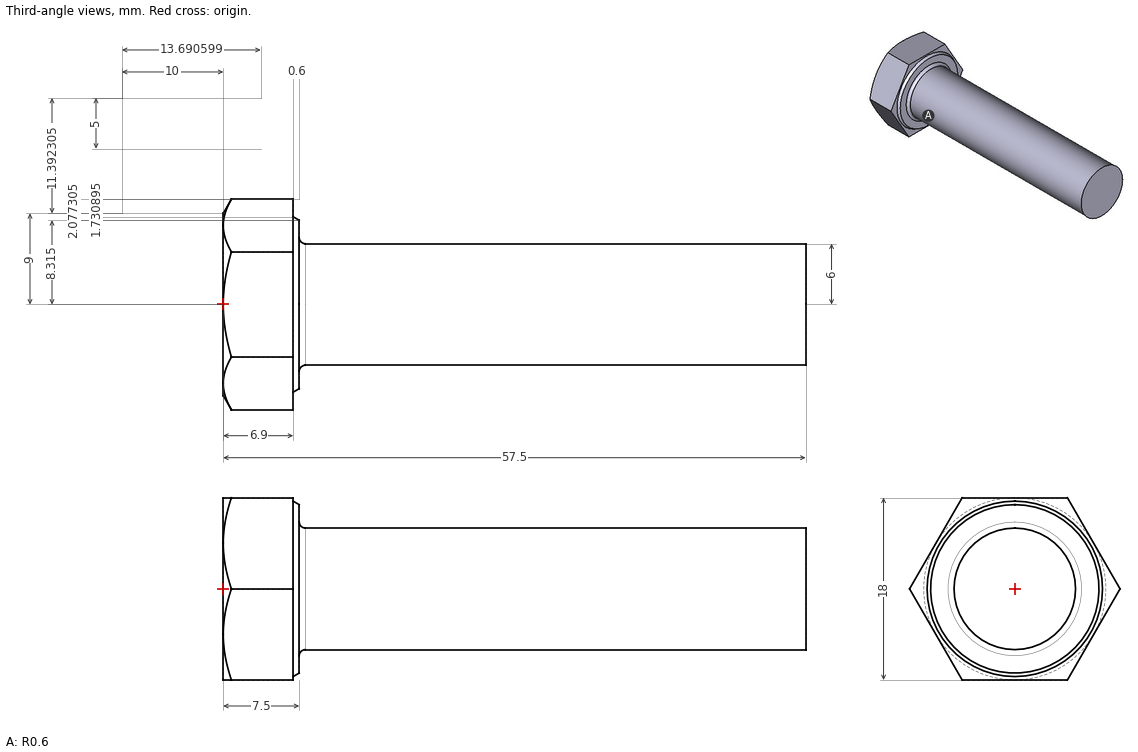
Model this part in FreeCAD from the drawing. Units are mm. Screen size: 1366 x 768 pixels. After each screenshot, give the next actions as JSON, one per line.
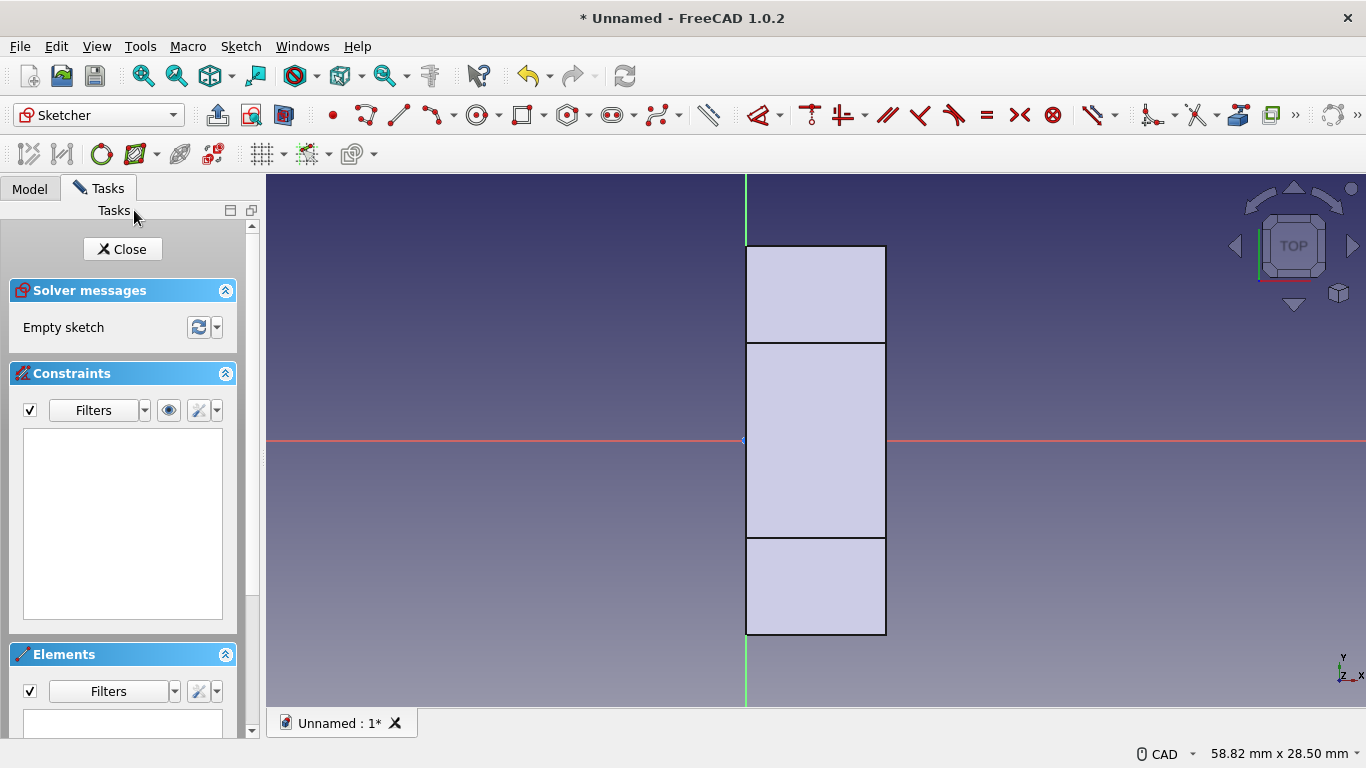
{"action": "left_click", "coordinate": [284, 116]}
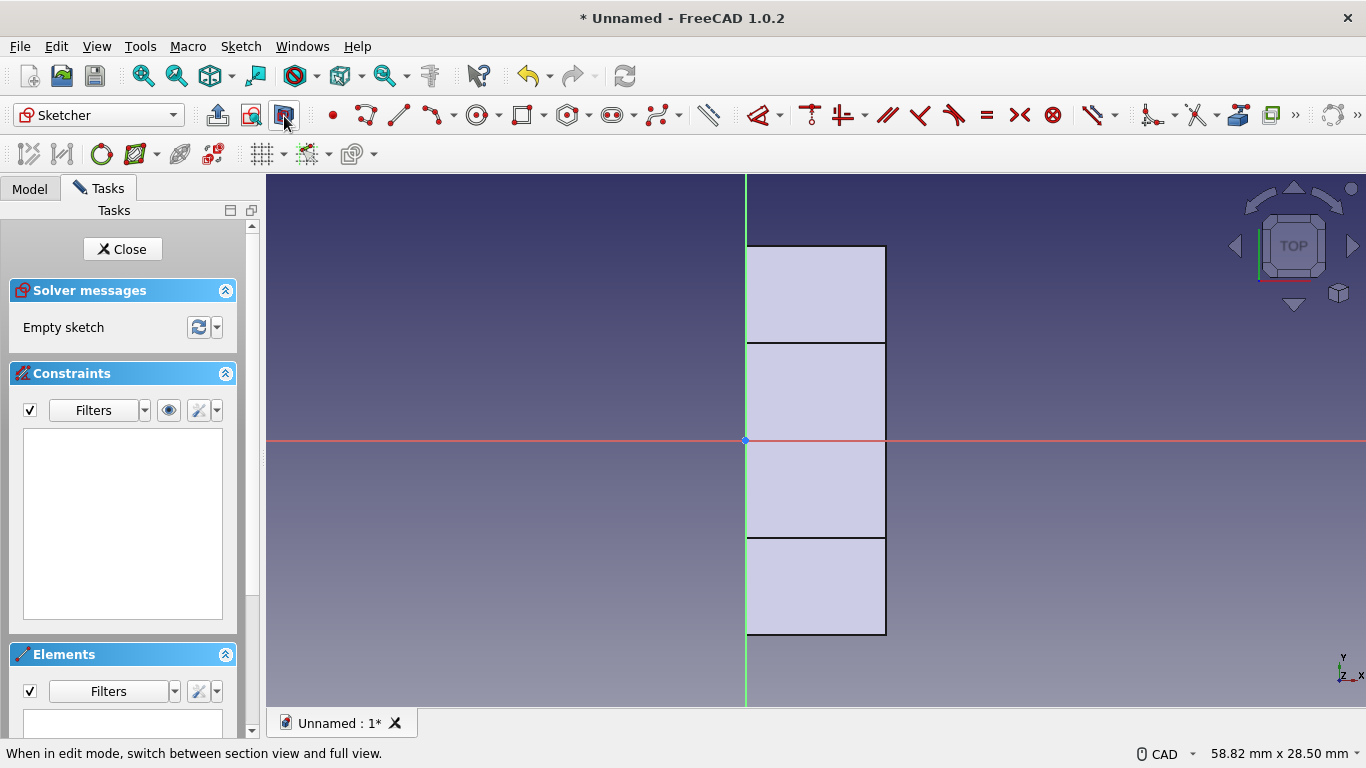
{"action": "scroll", "coordinate": [294, 509], "scroll_direction": "down", "scroll_amount": 3}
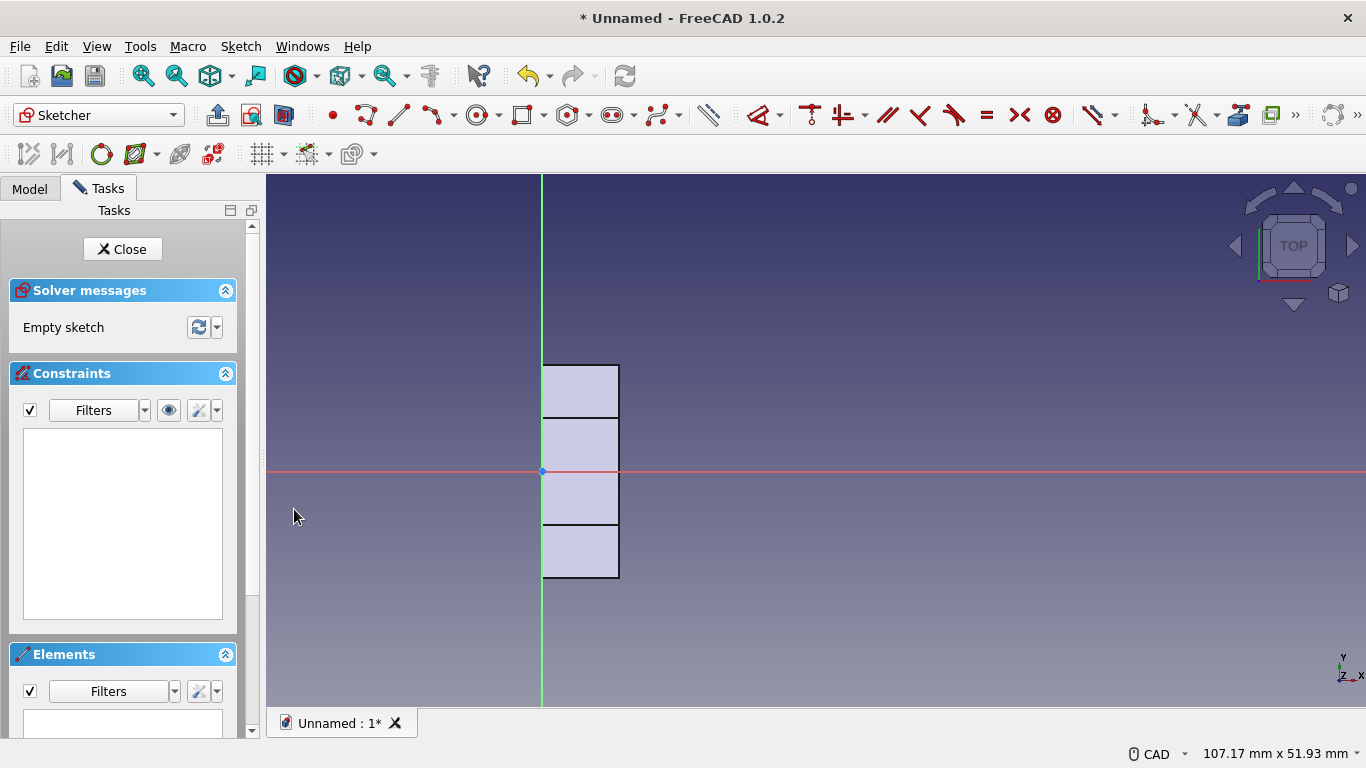
{"action": "left_click", "coordinate": [522, 116]}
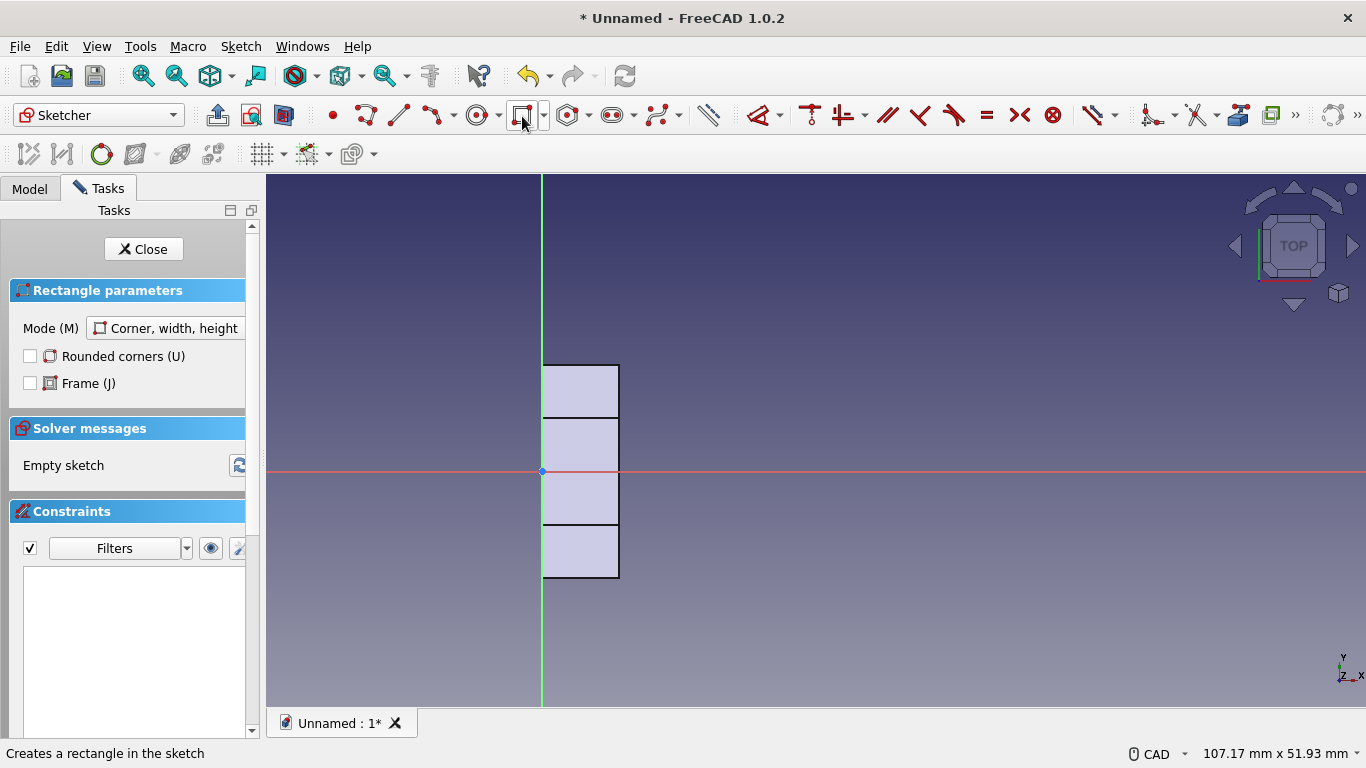
{"action": "left_click", "coordinate": [542, 472]}
{"action": "left_click", "coordinate": [1132, 410]}
{"action": "key", "text": "Escape"}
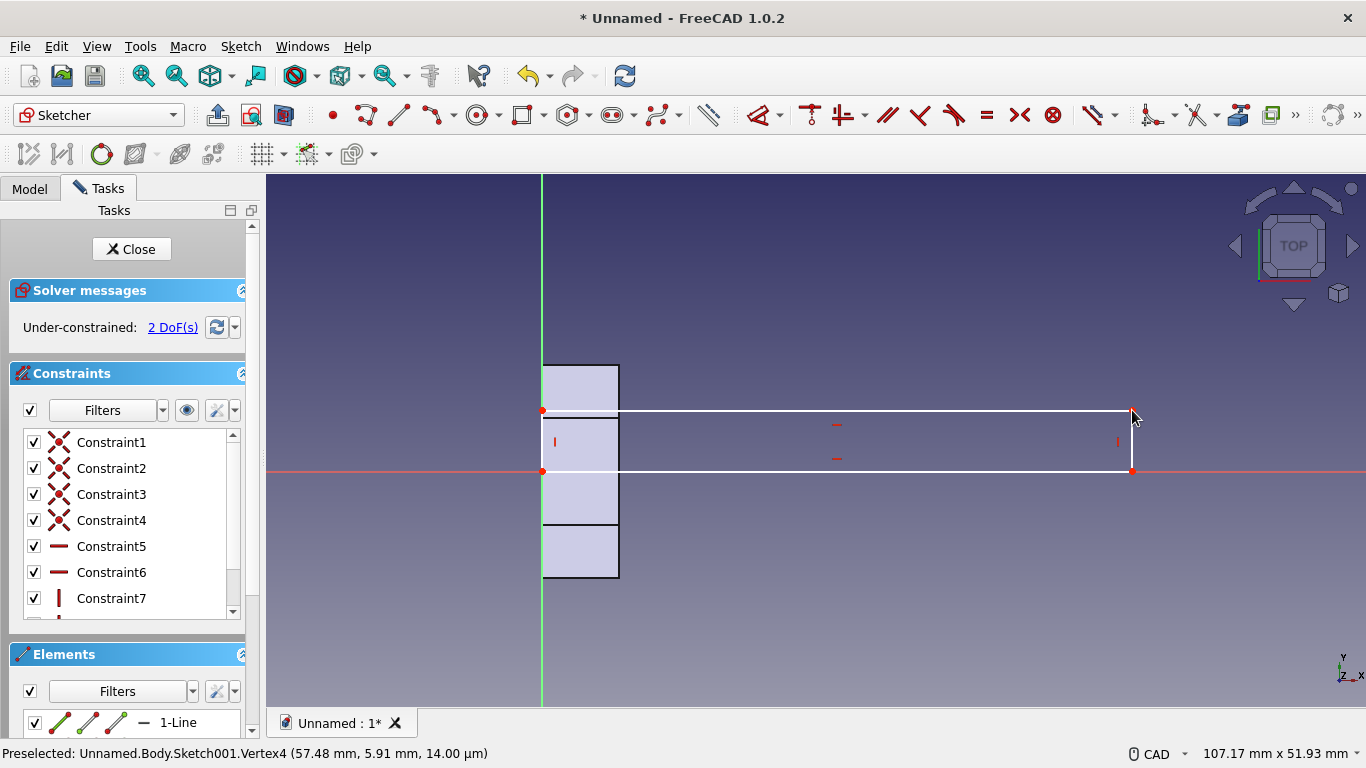
{"action": "left_click", "coordinate": [758, 116]}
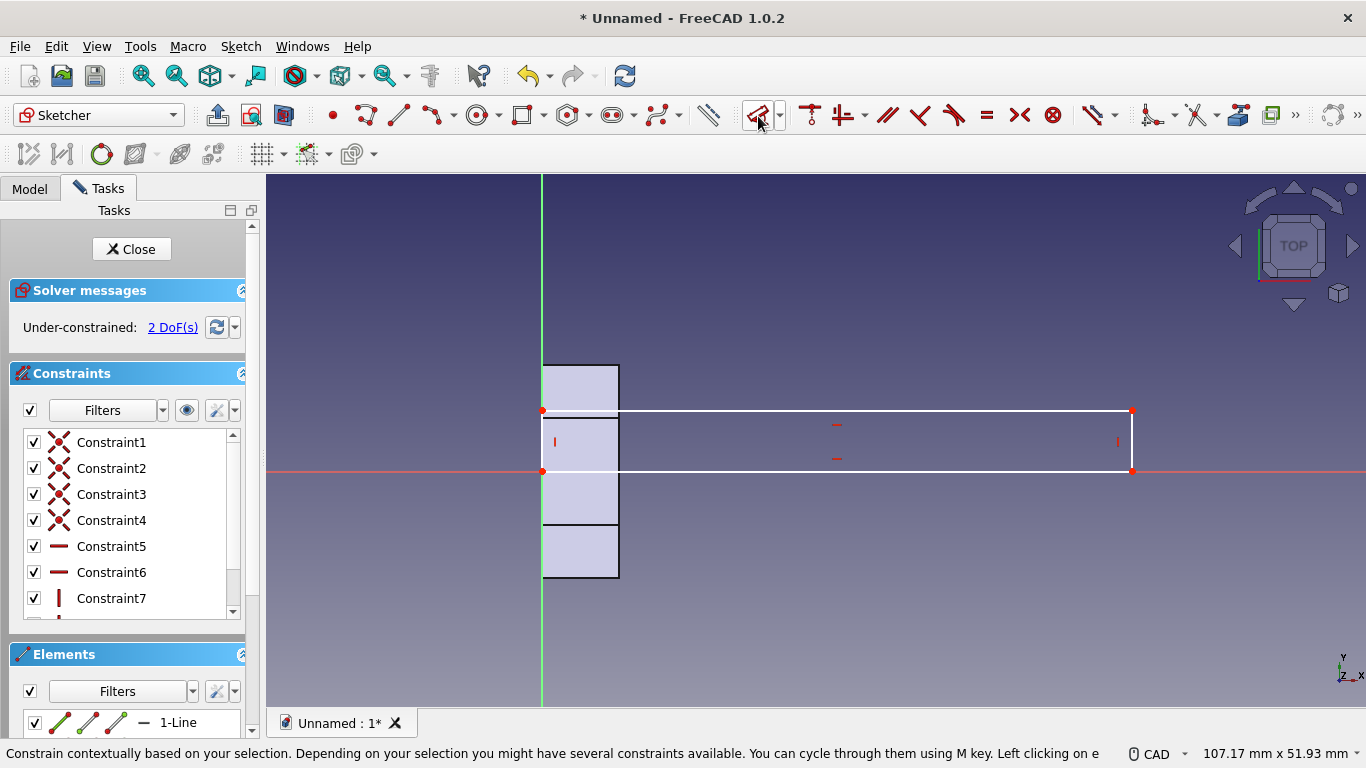
{"action": "left_click", "coordinate": [1132, 453]}
{"action": "left_click", "coordinate": [1166, 441]}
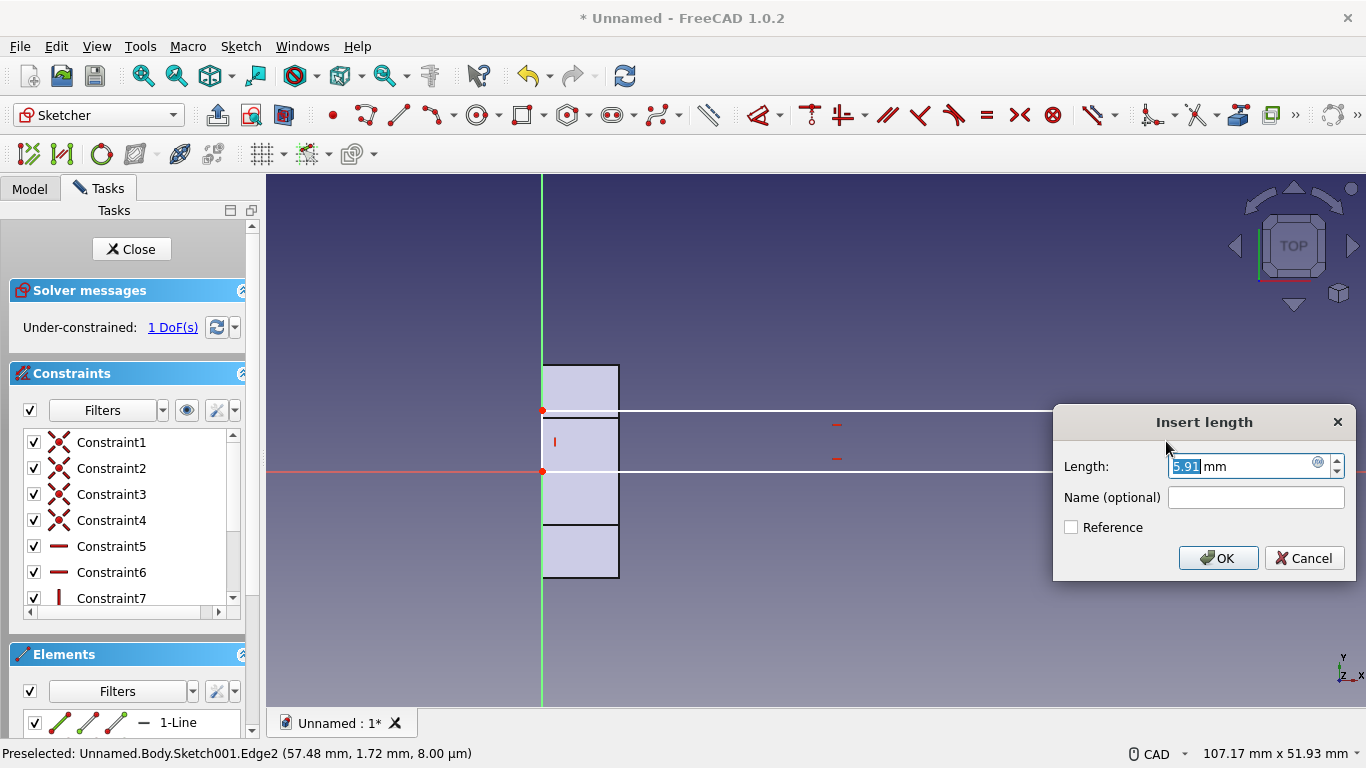
{"action": "type", "text": "6"}
{"action": "key", "text": "Return"}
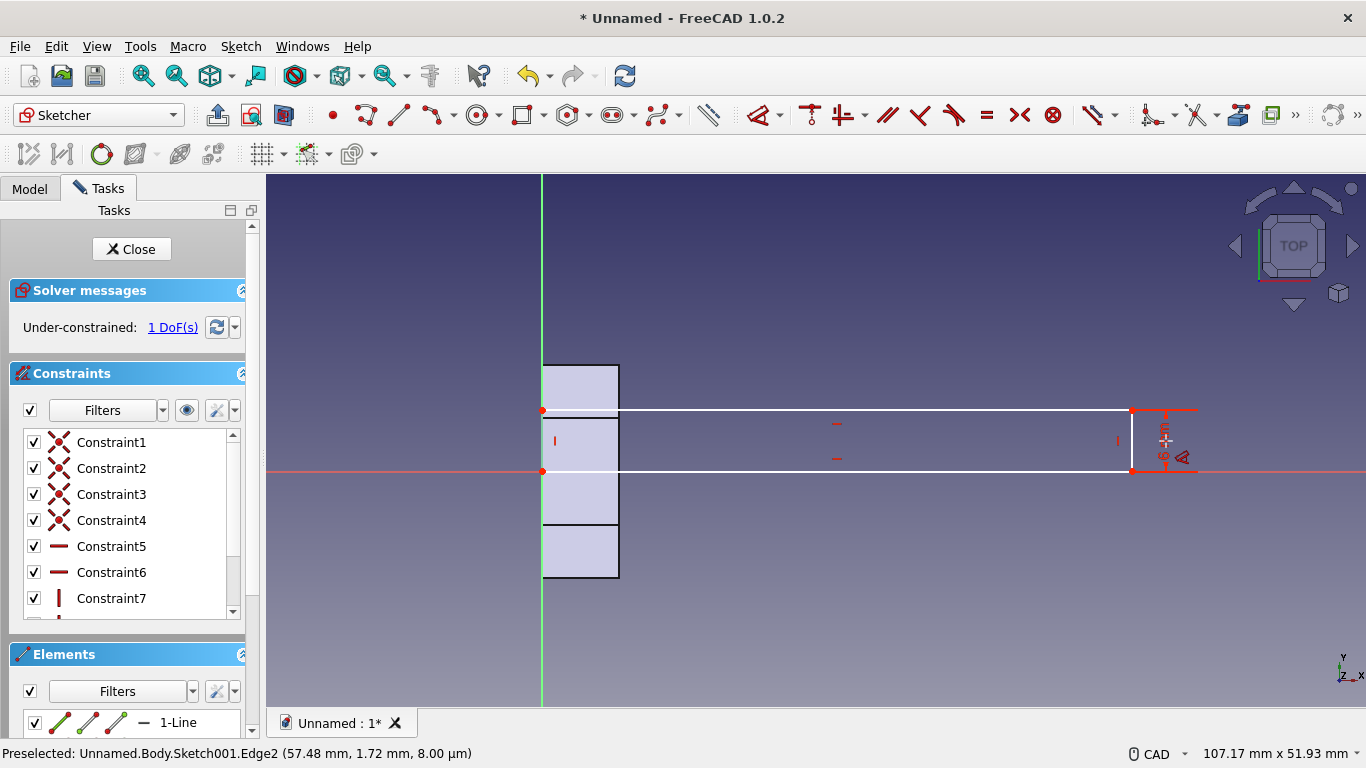
{"action": "left_click", "coordinate": [719, 472]}
{"action": "left_click", "coordinate": [837, 506]}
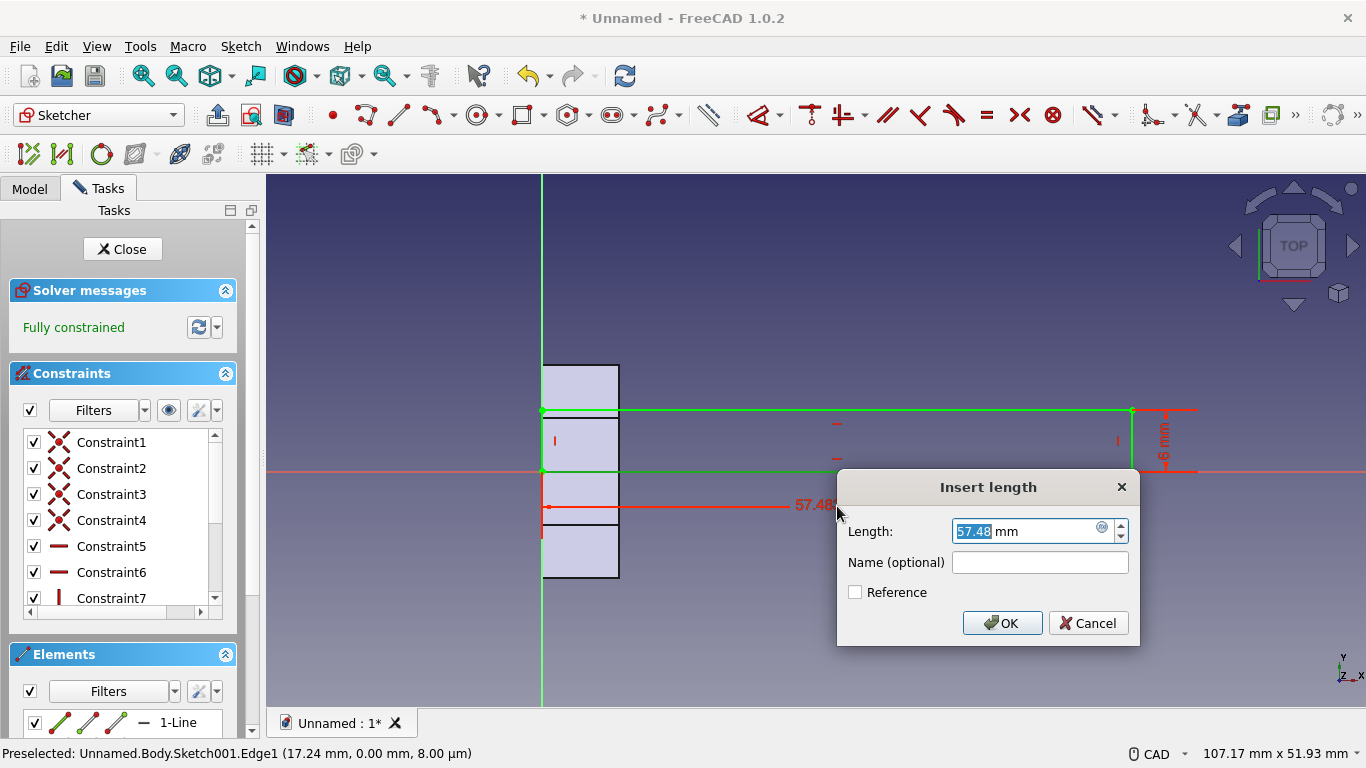
{"action": "type", "text": "57.5"}
{"action": "key", "text": "Return"}
{"action": "key", "text": "Escape"}